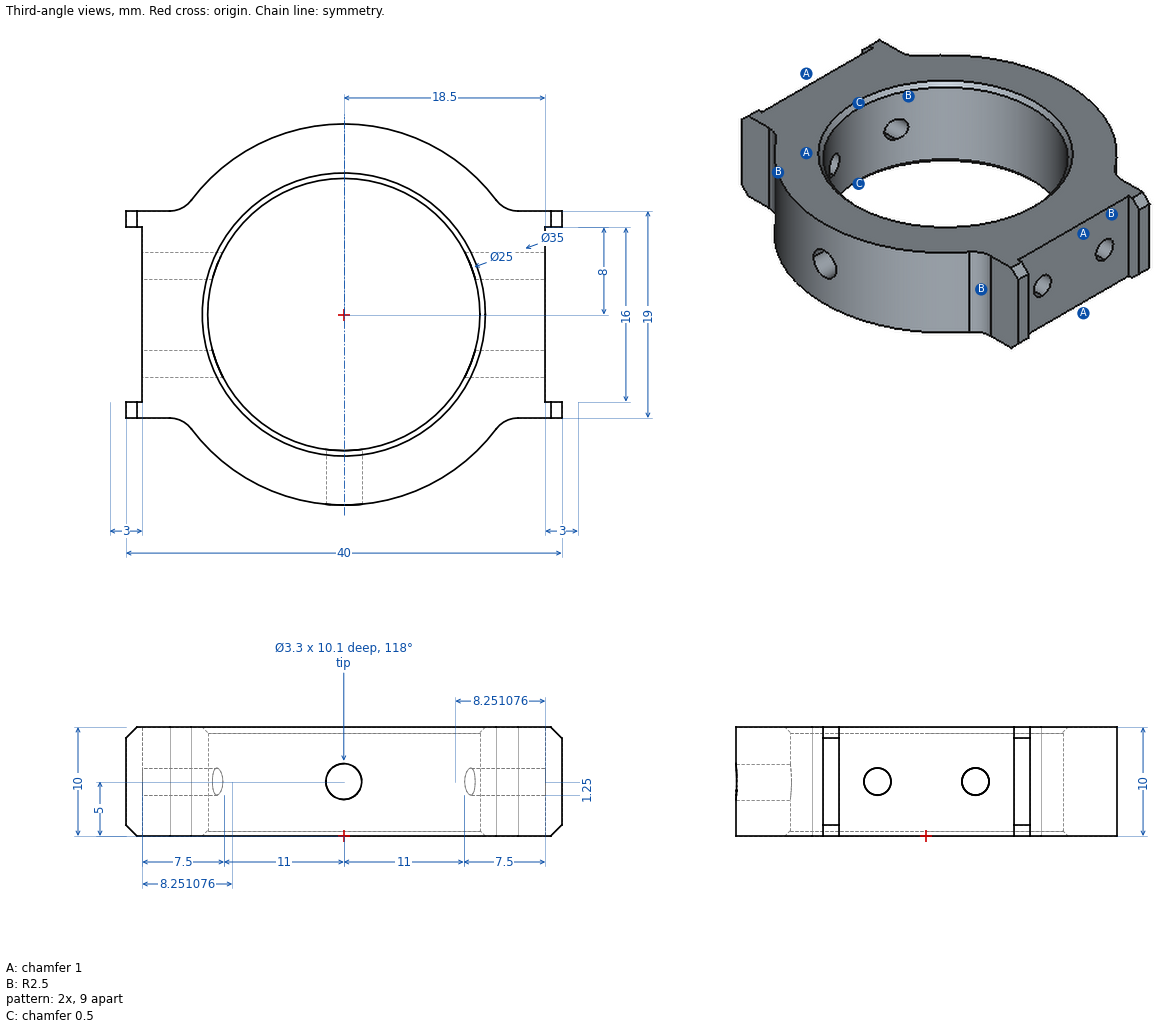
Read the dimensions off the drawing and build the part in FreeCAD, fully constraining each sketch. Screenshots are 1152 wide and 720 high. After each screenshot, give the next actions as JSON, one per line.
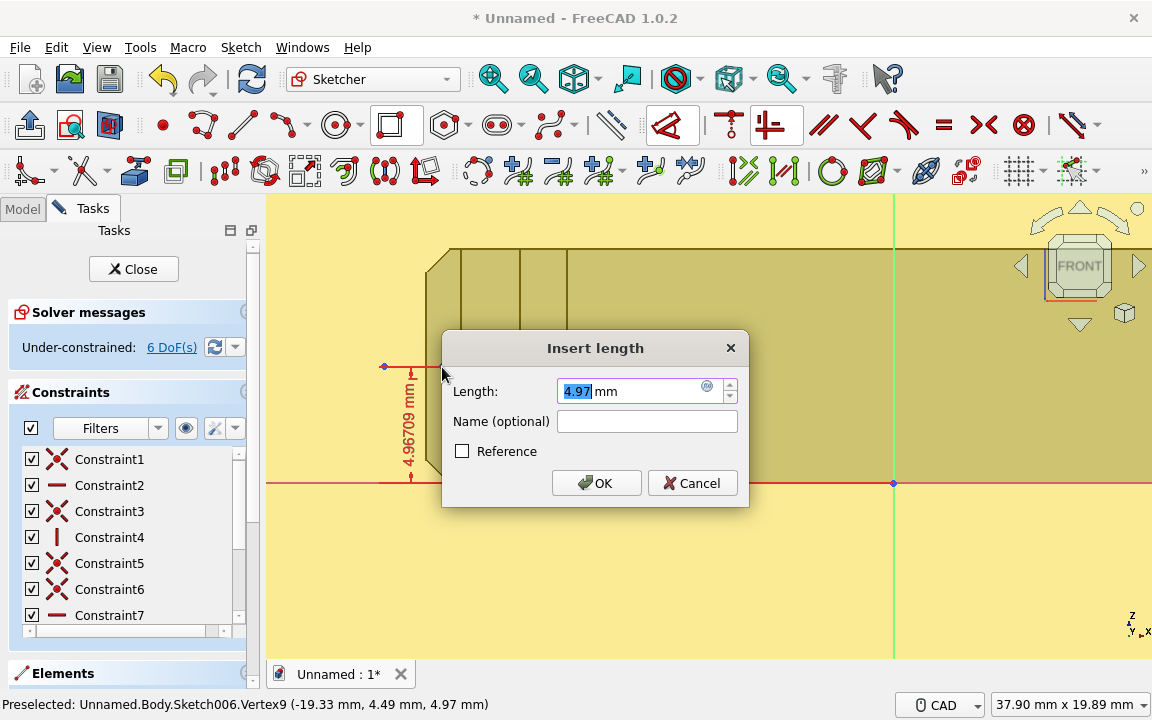
{"action": "type", "text": "5"}
{"action": "key", "text": "Return"}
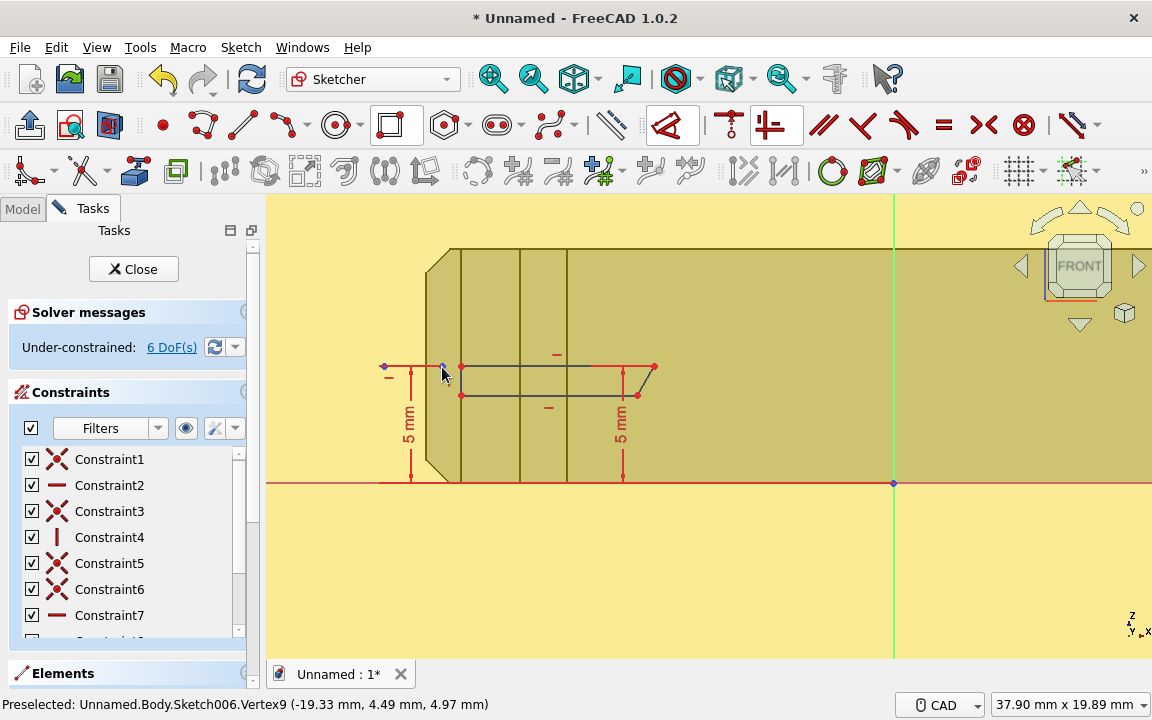
{"action": "left_click", "coordinate": [584, 396]}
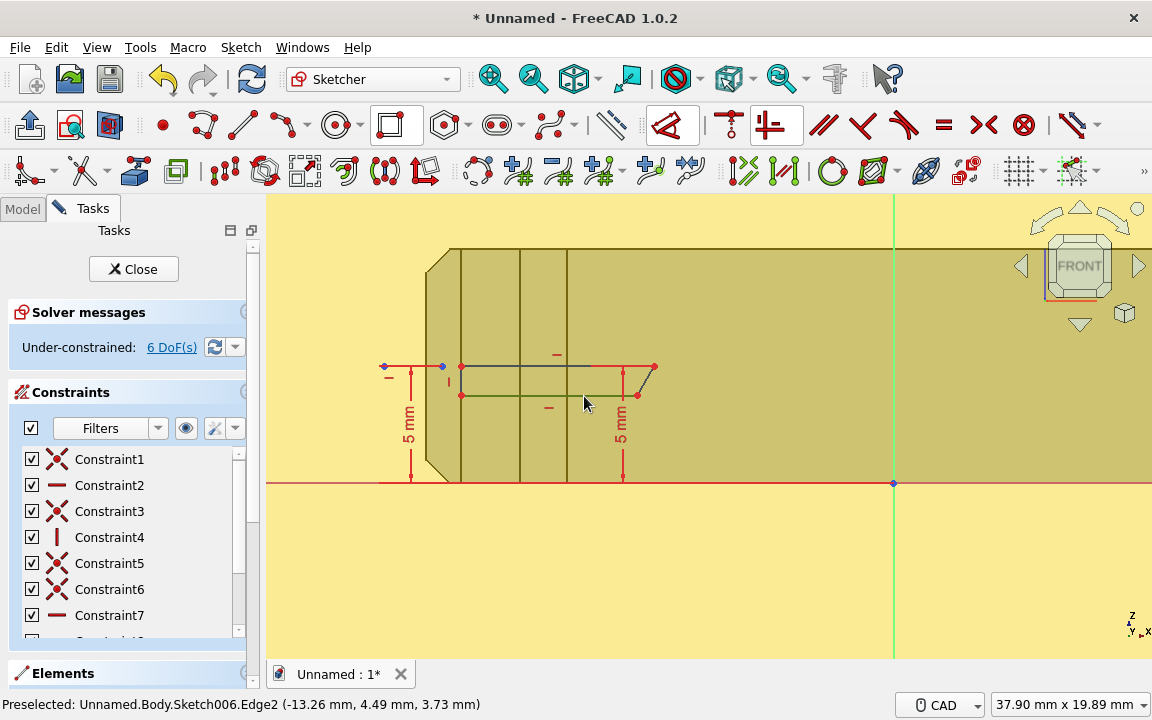
{"action": "left_click", "coordinate": [694, 126]}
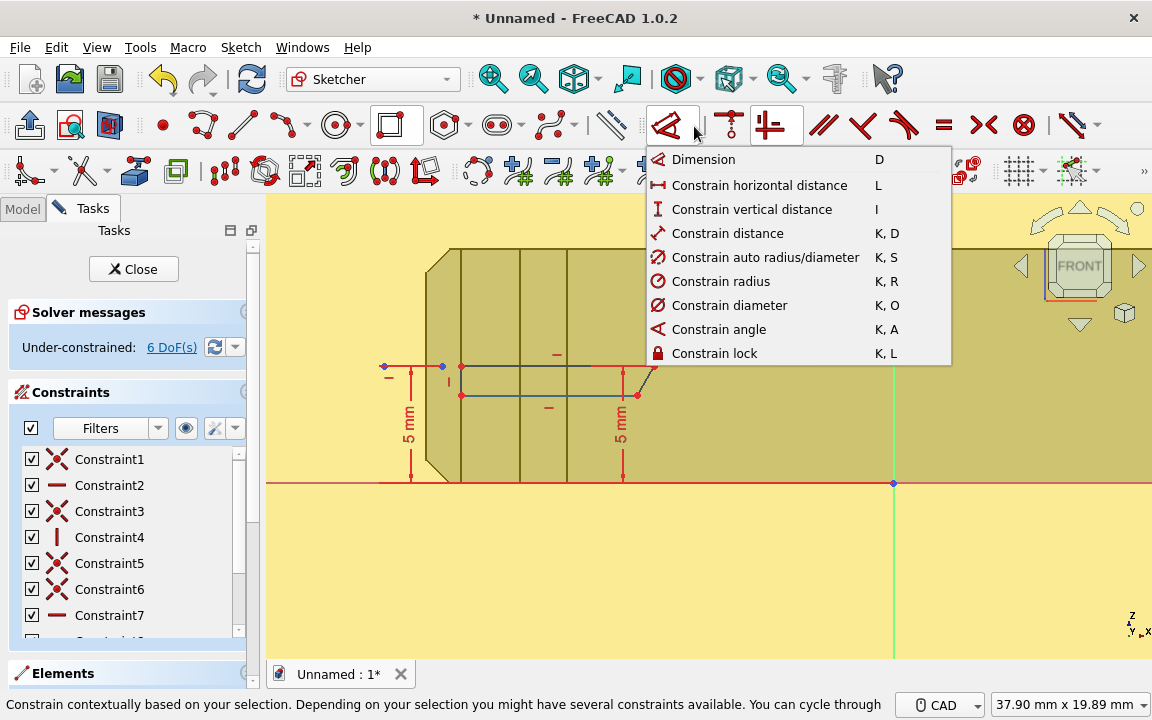
{"action": "left_click", "coordinate": [799, 185]}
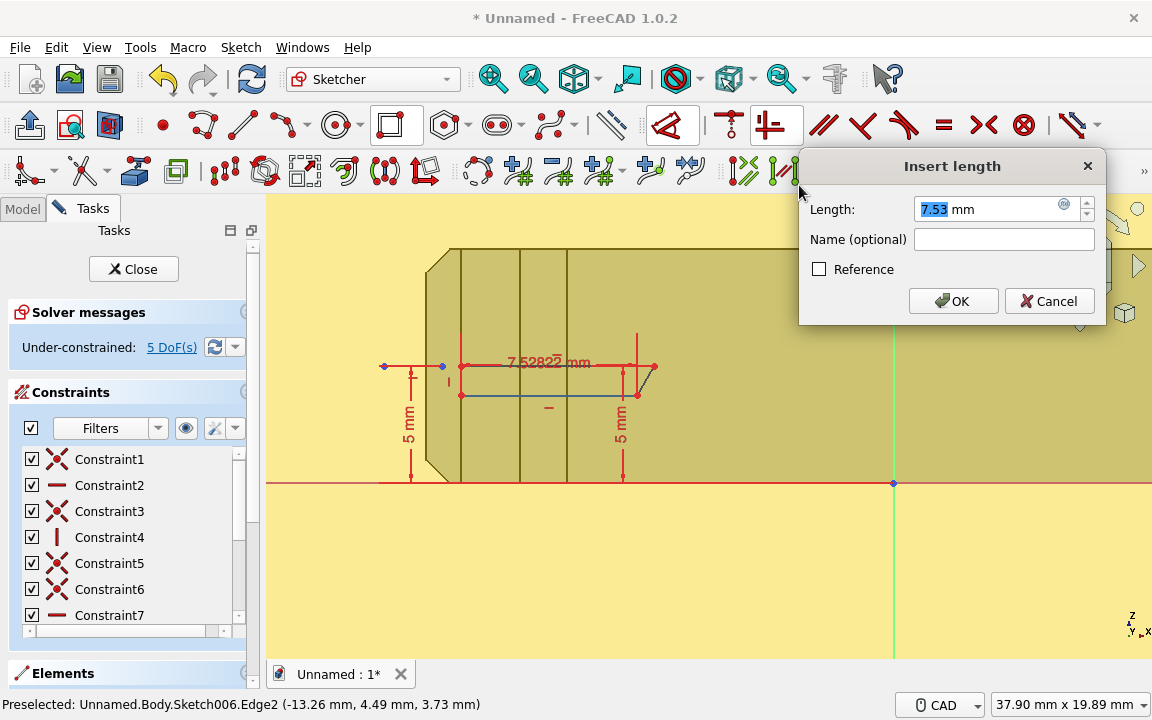
{"action": "type", "text": "7.5"}
{"action": "key", "text": "Return"}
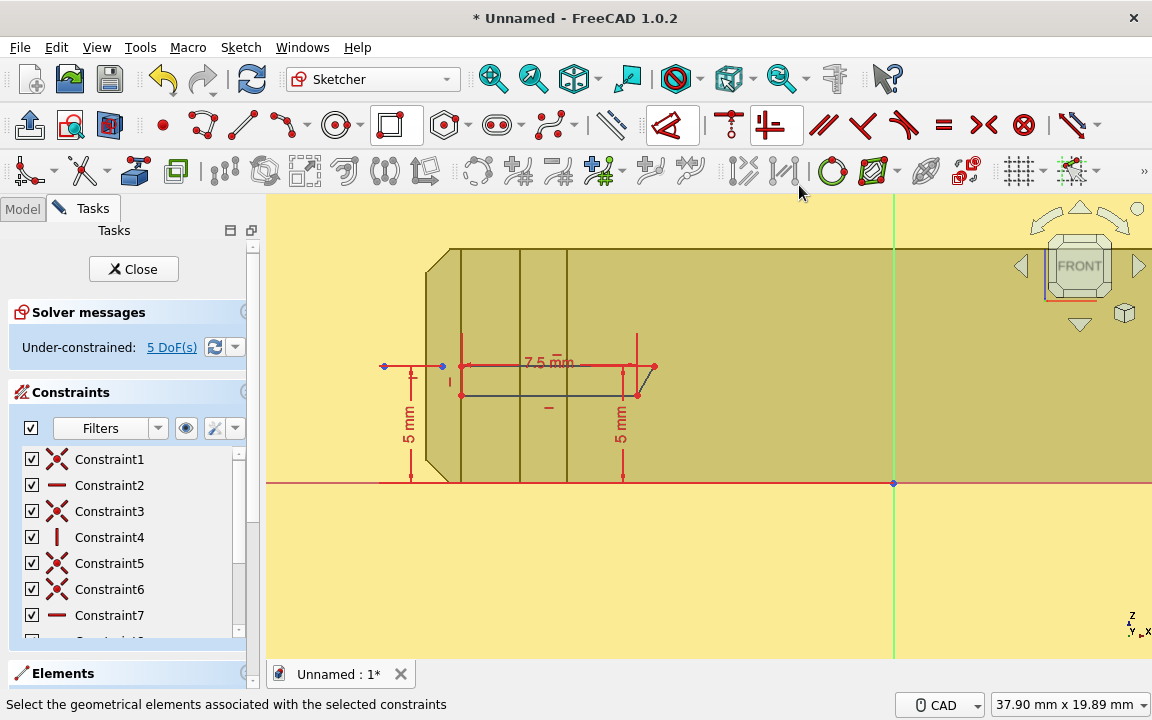
{"action": "left_click", "coordinate": [637, 396]}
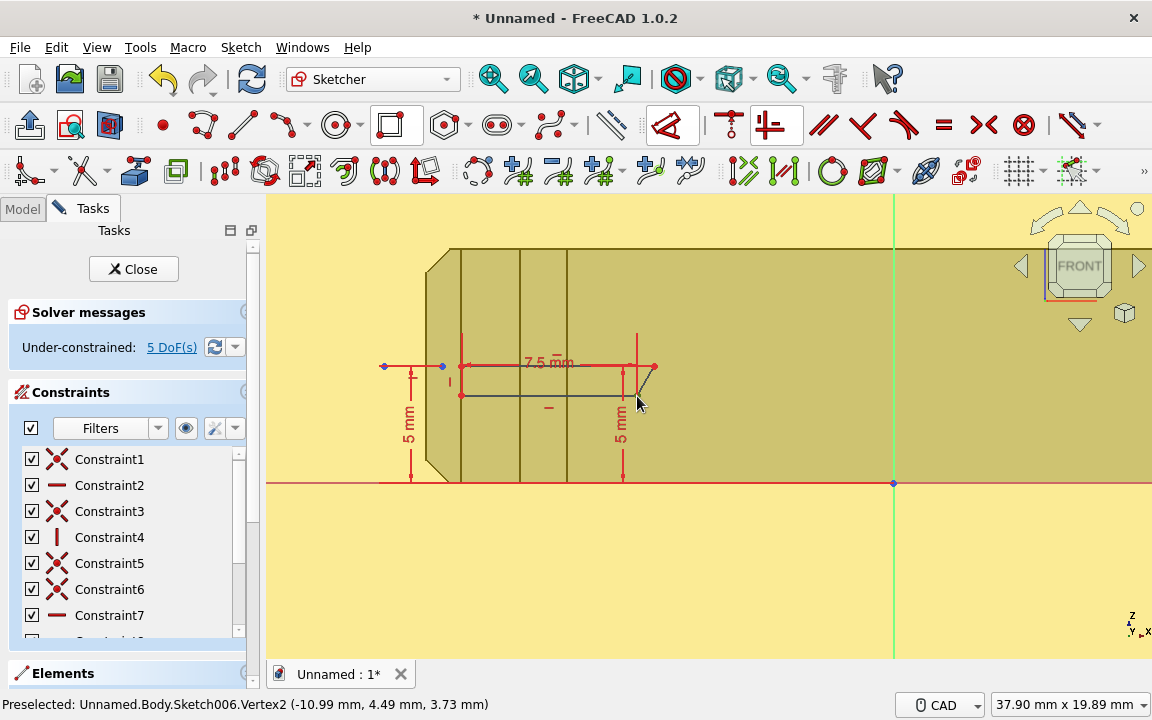
{"action": "left_click", "coordinate": [694, 126]}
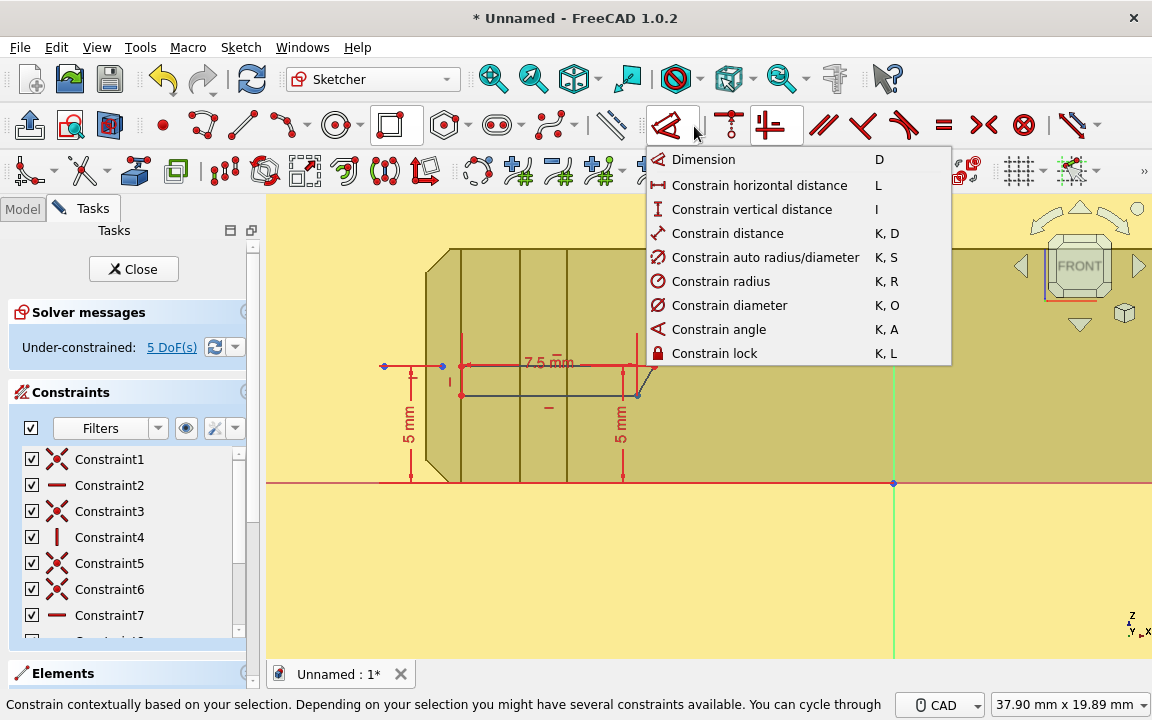
{"action": "left_click", "coordinate": [799, 185]}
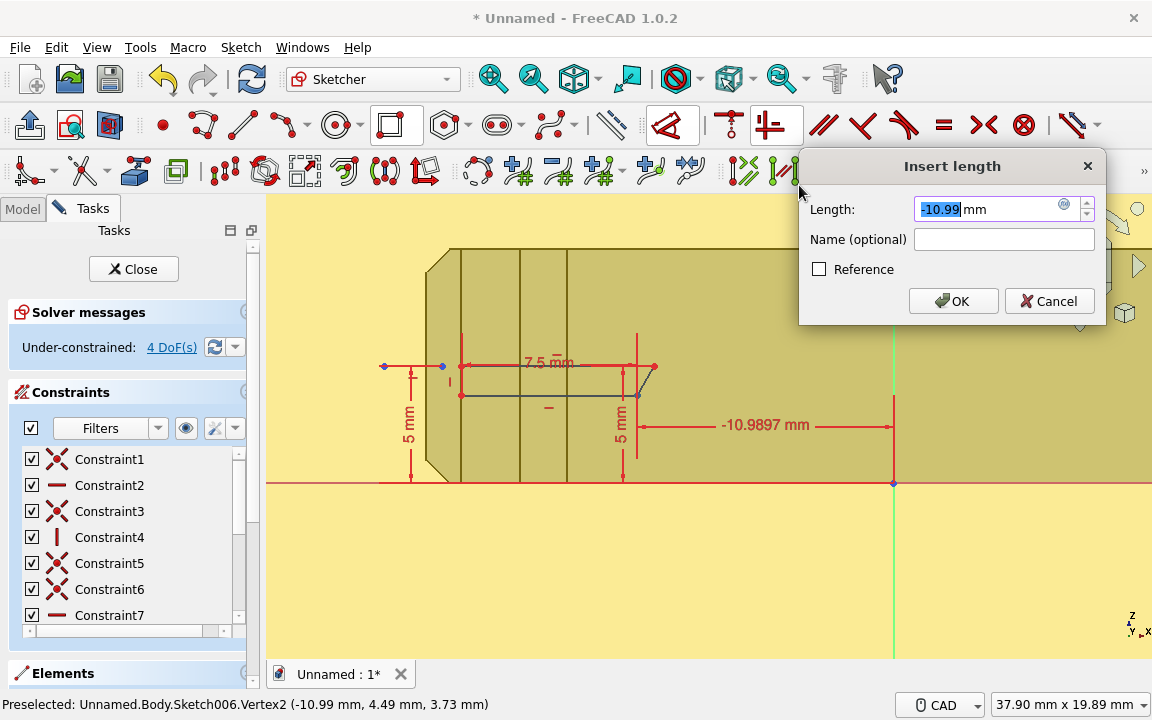
{"action": "type", "text": "-11"}
{"action": "key", "text": "Return"}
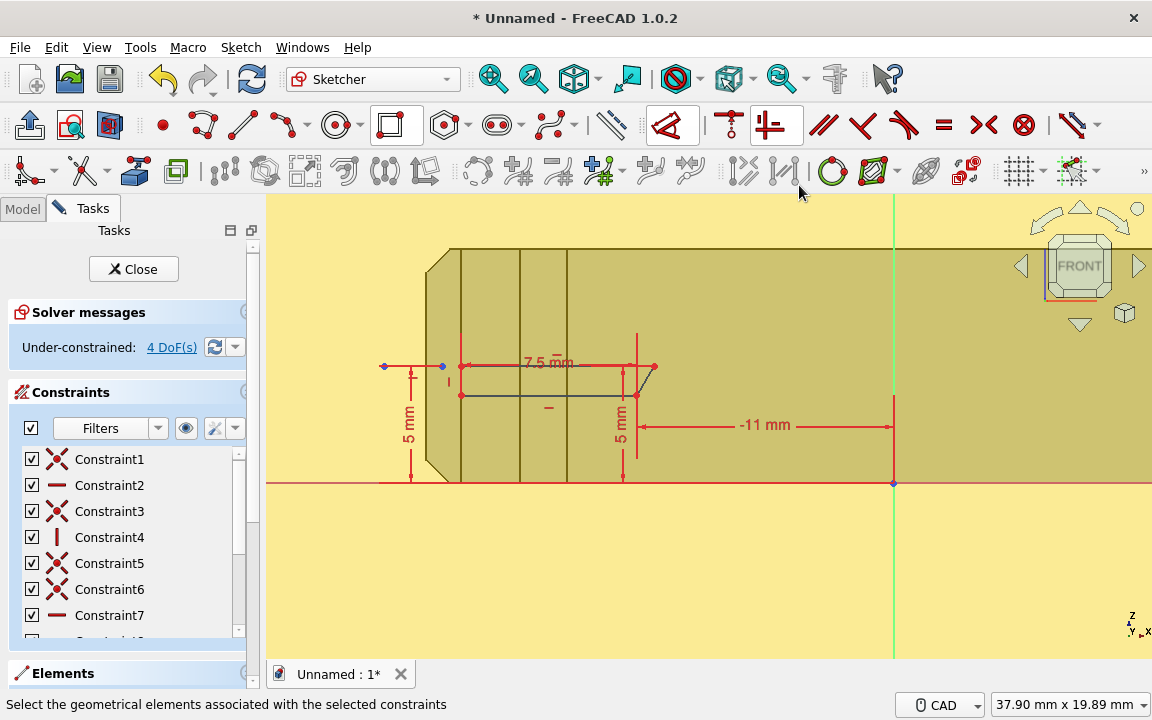
{"action": "scroll", "coordinate": [461, 384], "scroll_direction": "up", "scroll_amount": 2}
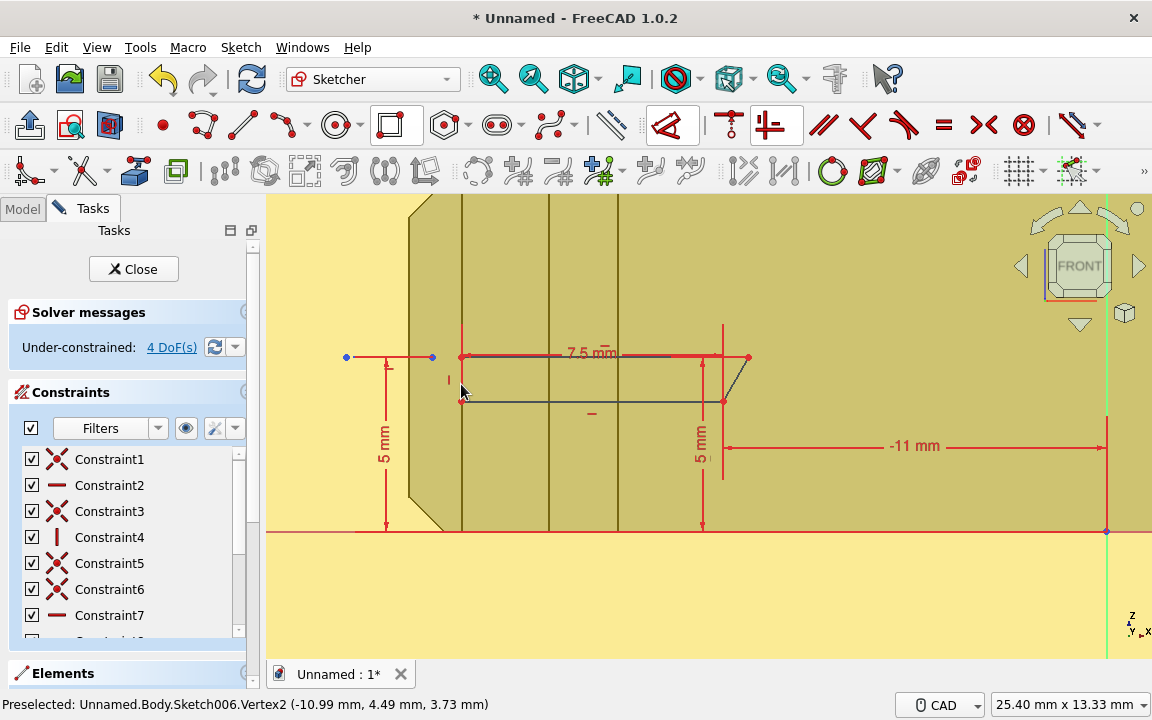
{"action": "left_click", "coordinate": [462, 384]}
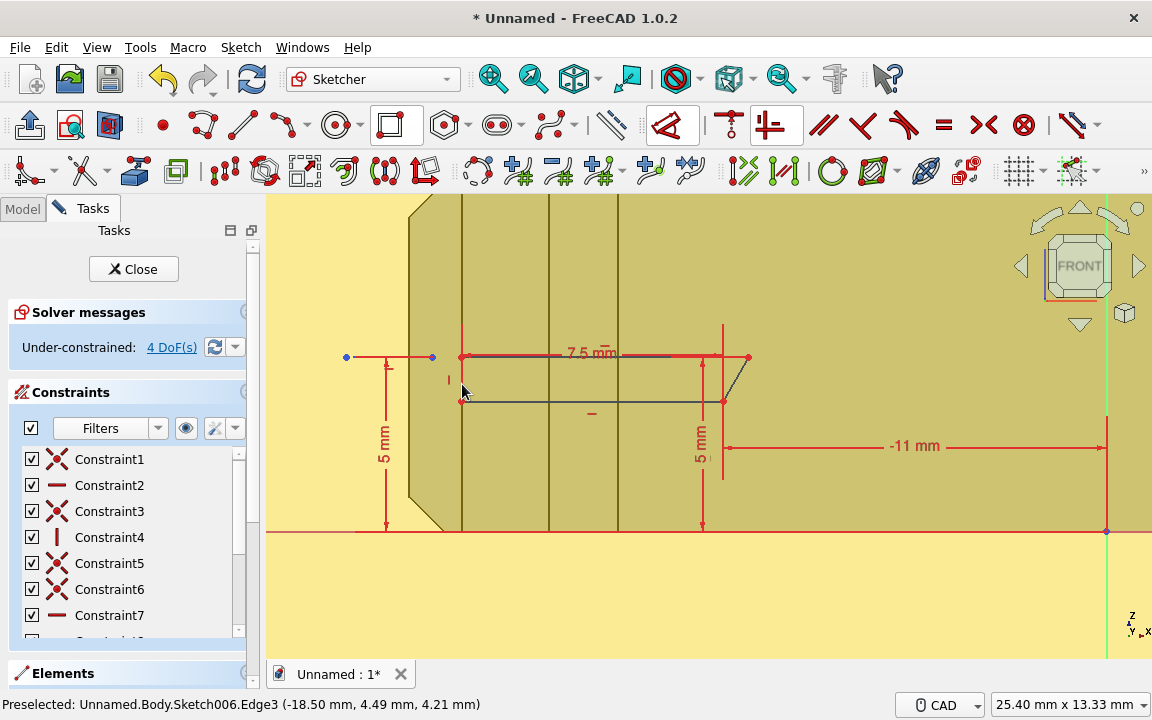
{"action": "left_click", "coordinate": [694, 126]}